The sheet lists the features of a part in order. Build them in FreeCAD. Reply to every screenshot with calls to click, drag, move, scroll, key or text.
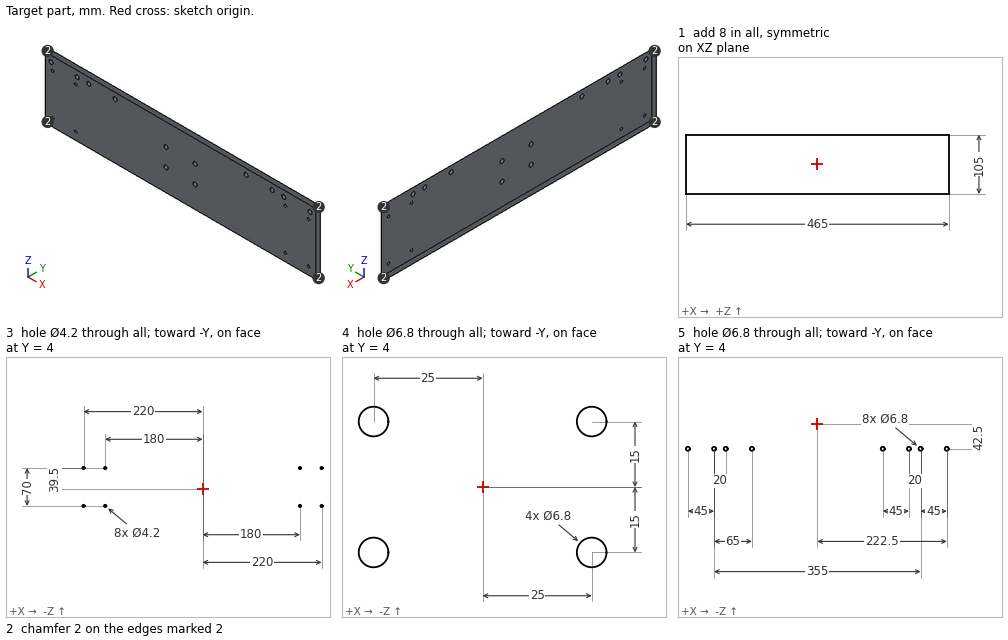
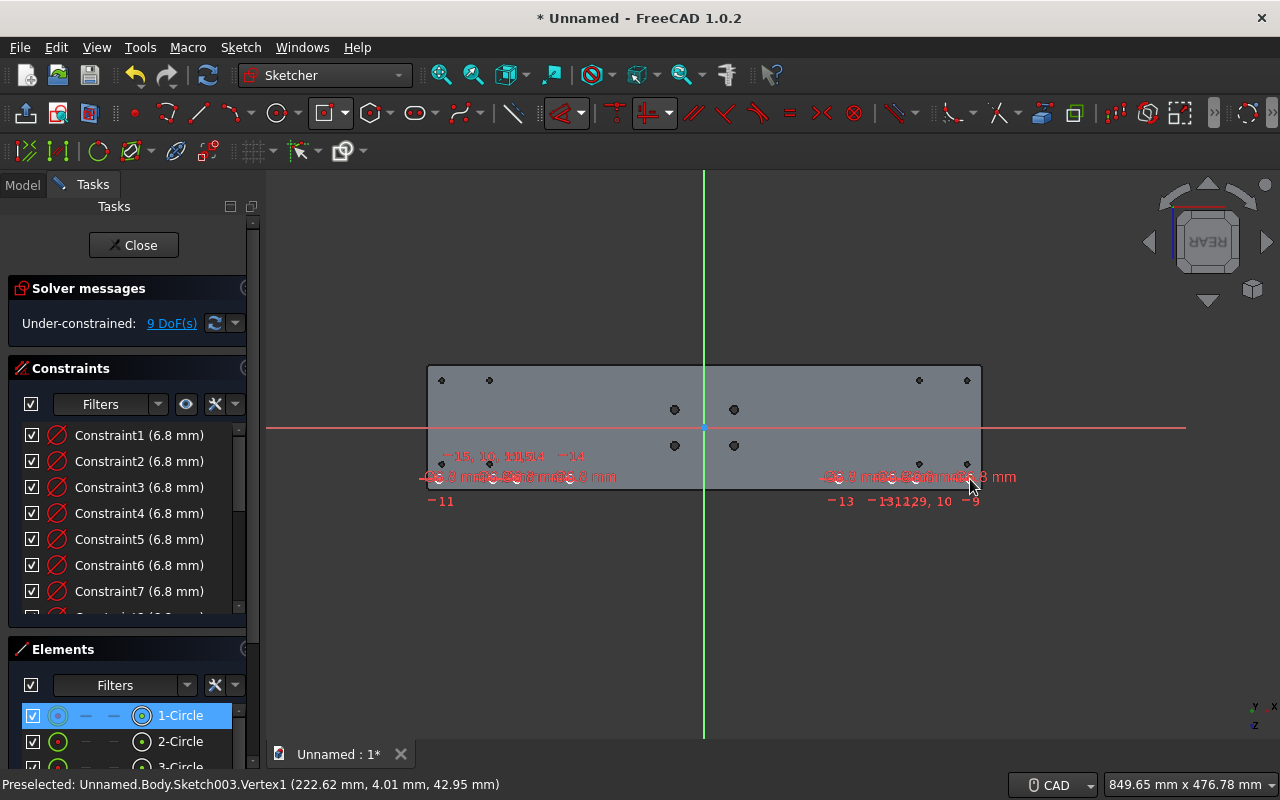
click(916, 479)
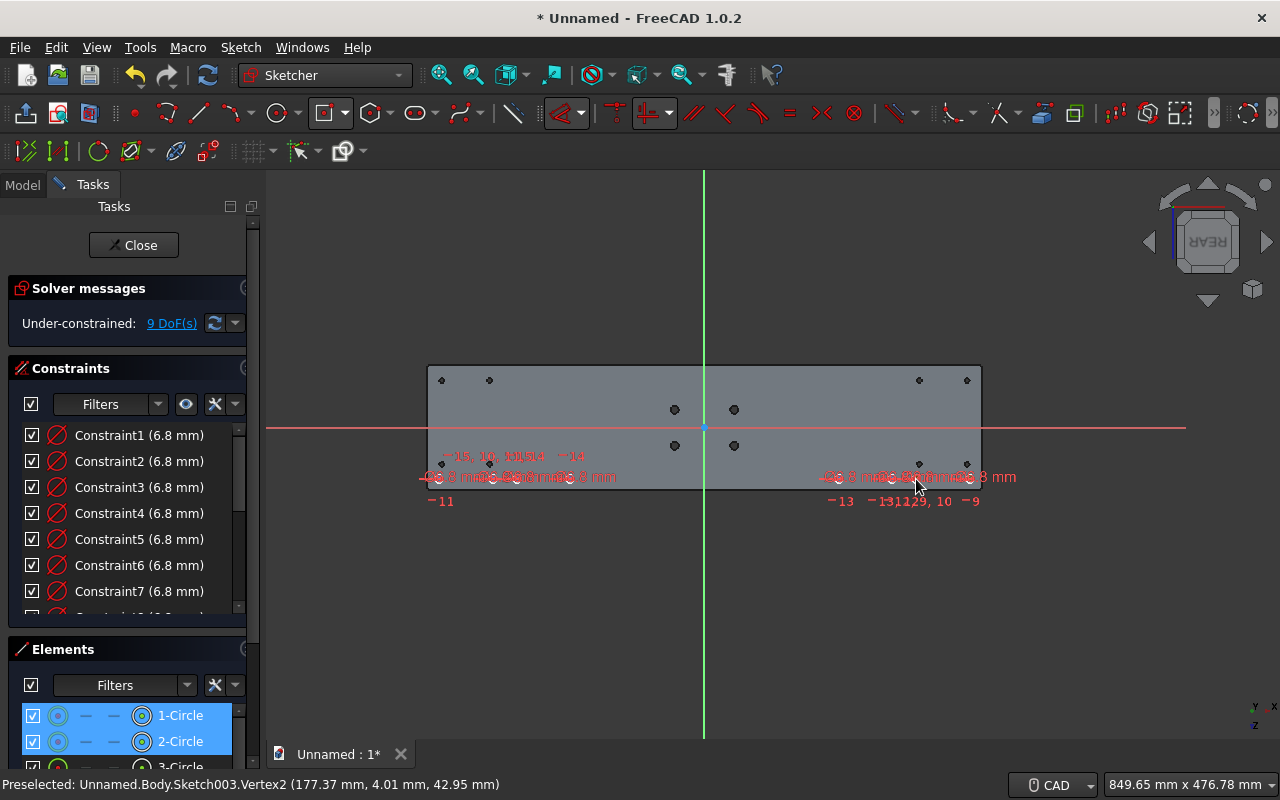
key(l)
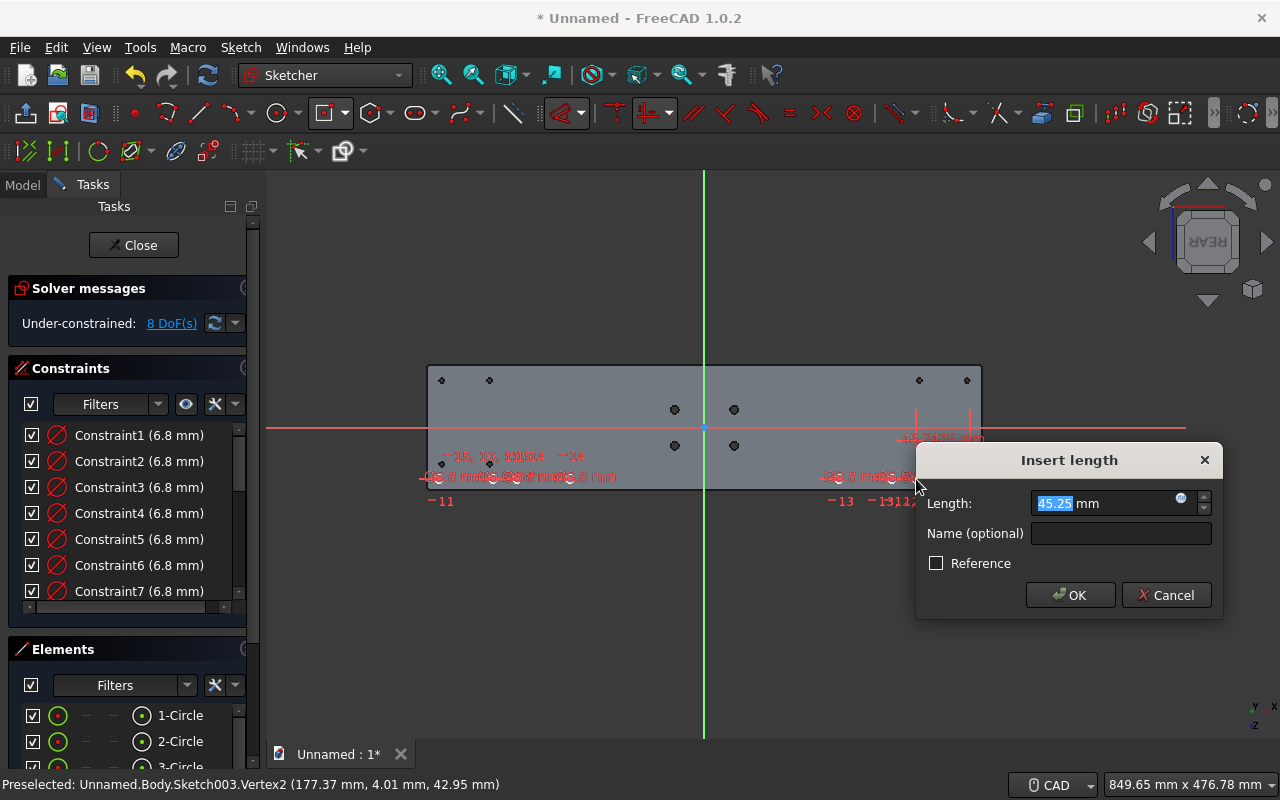
text(45)
key(Return)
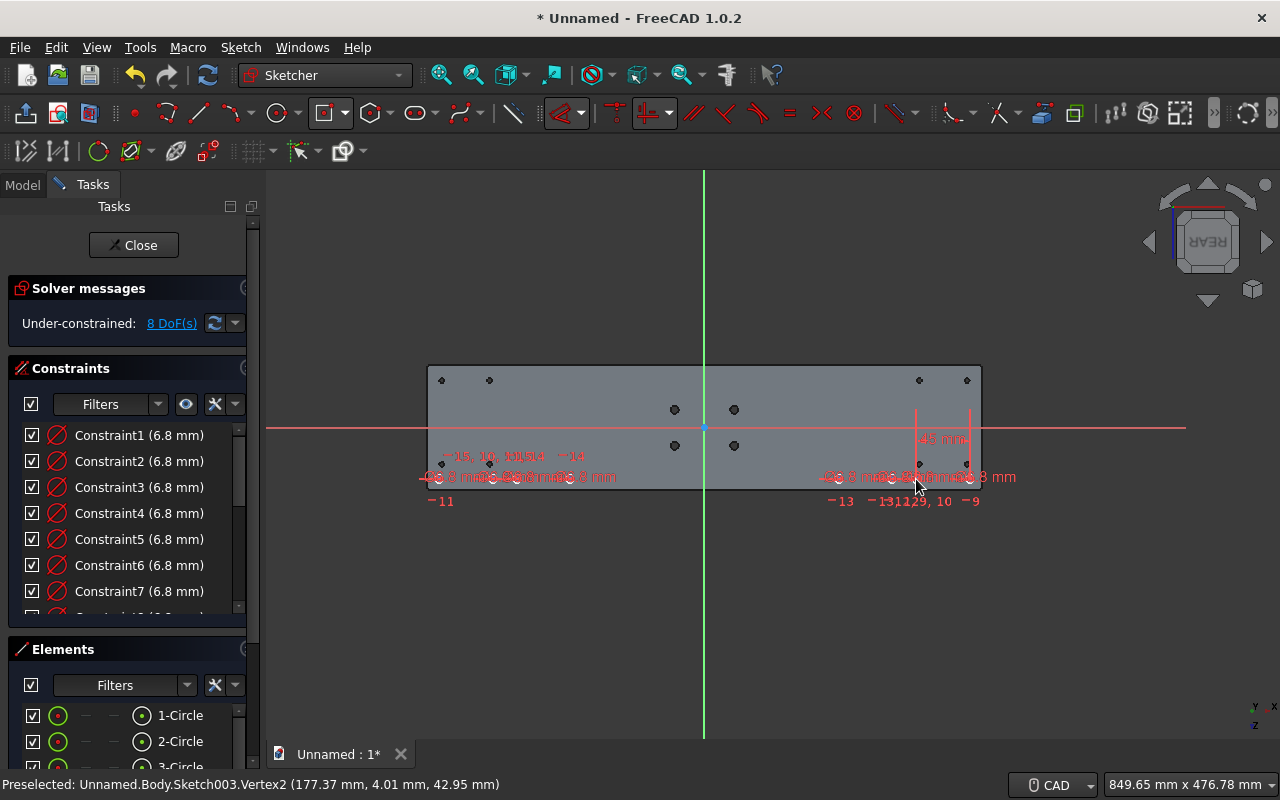
click(493, 479)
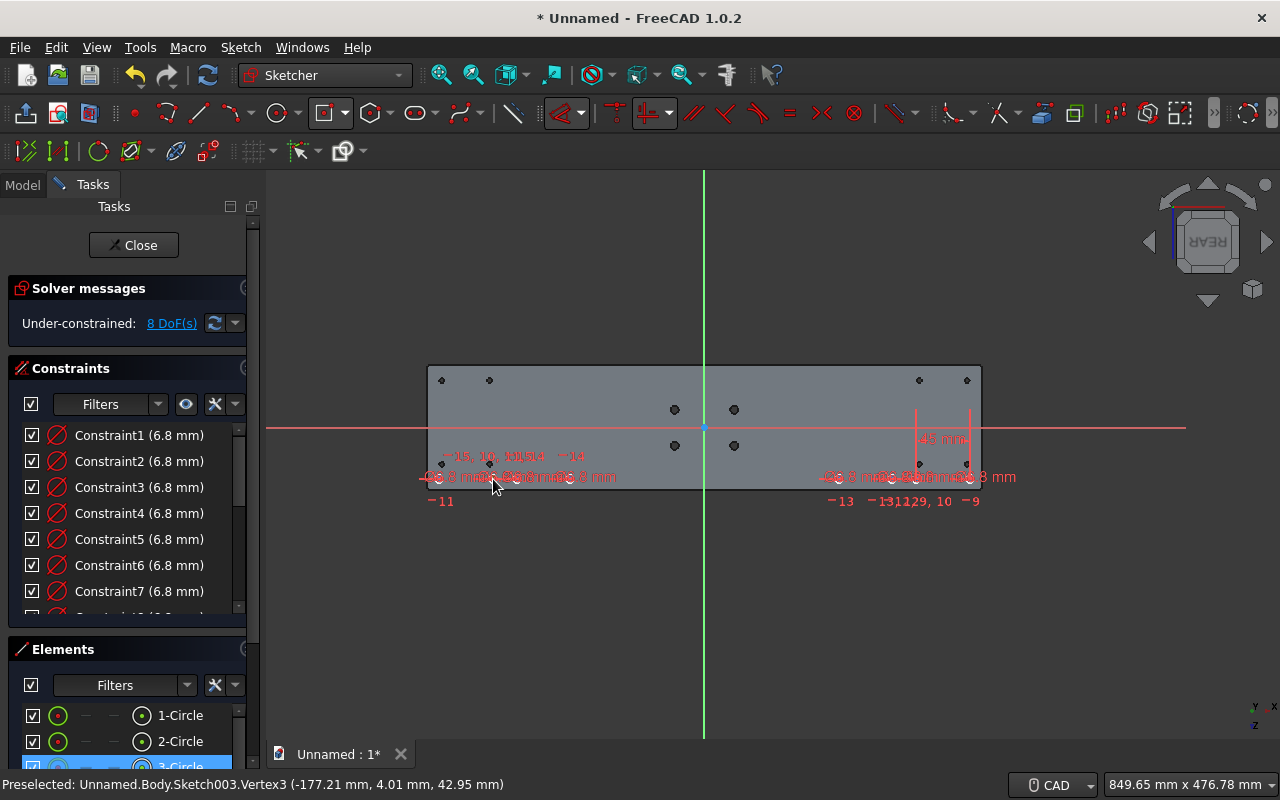
click(439, 479)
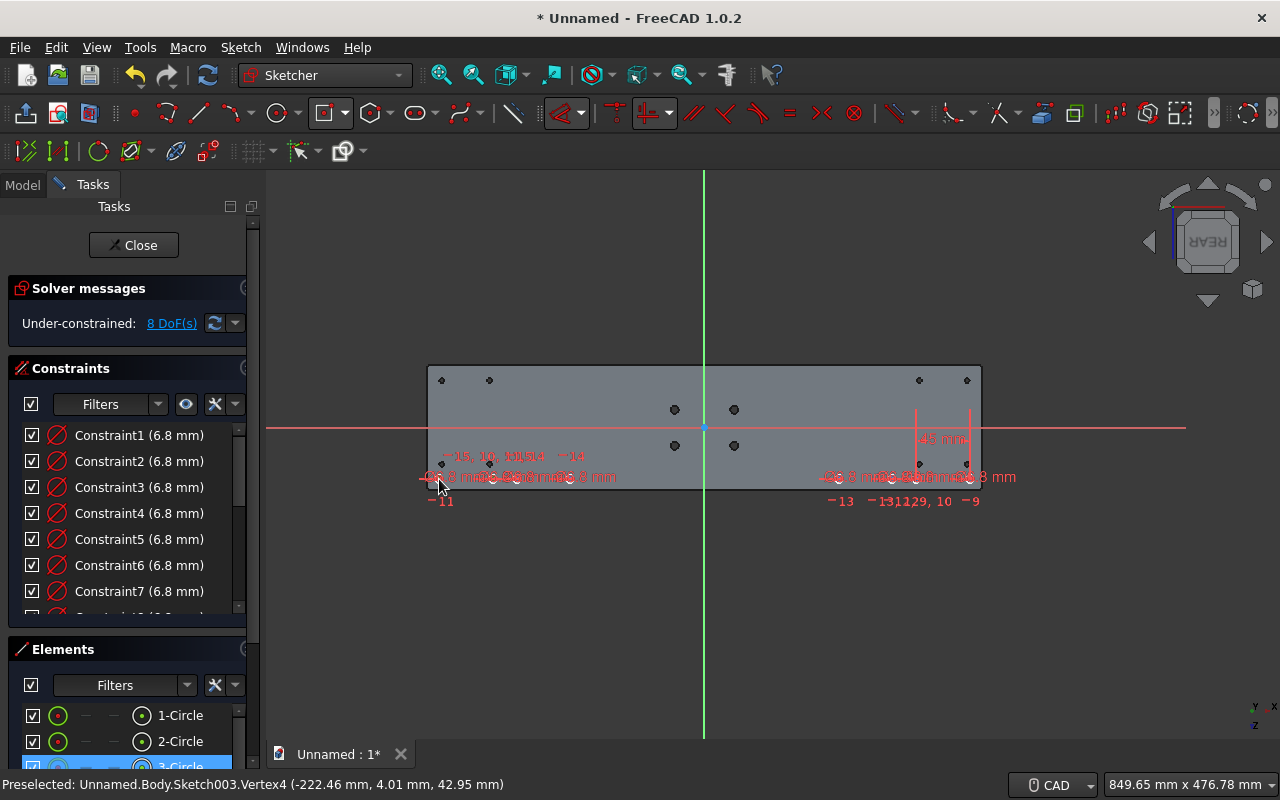
click(584, 114)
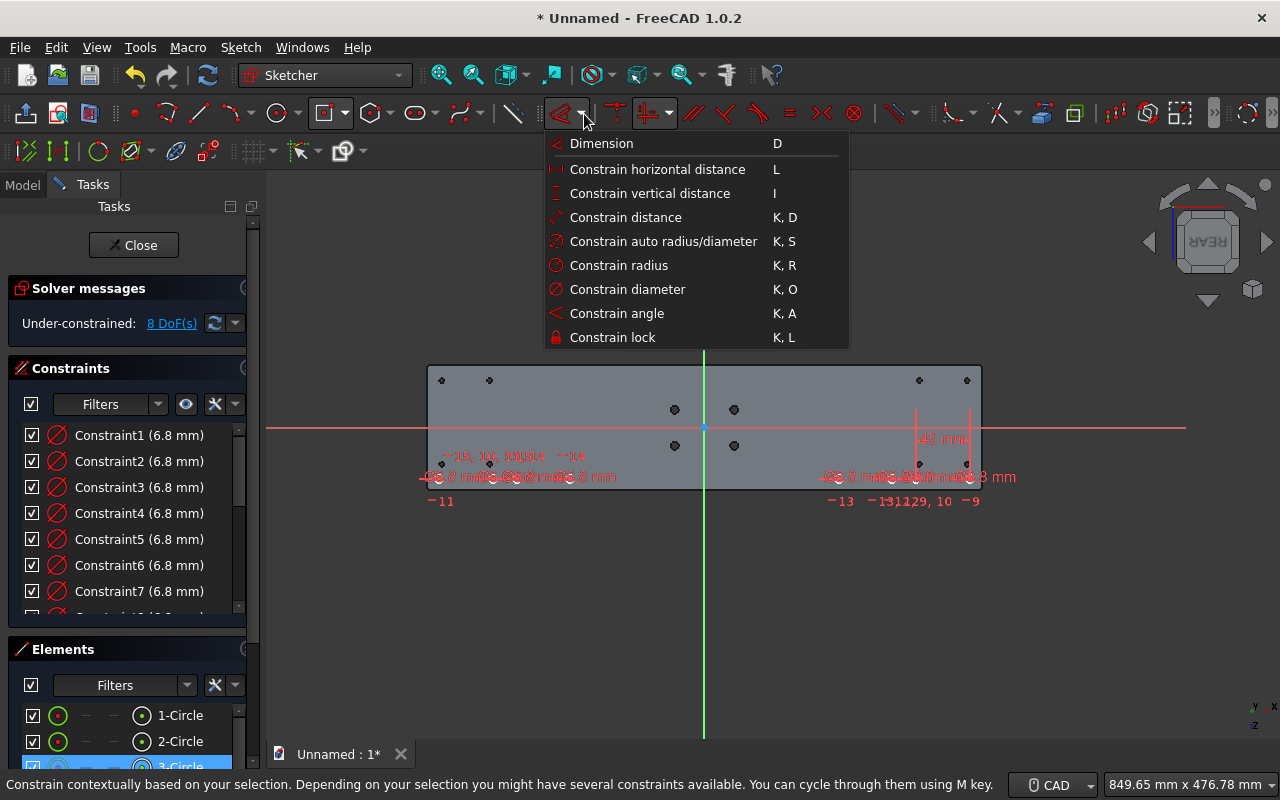
click(697, 169)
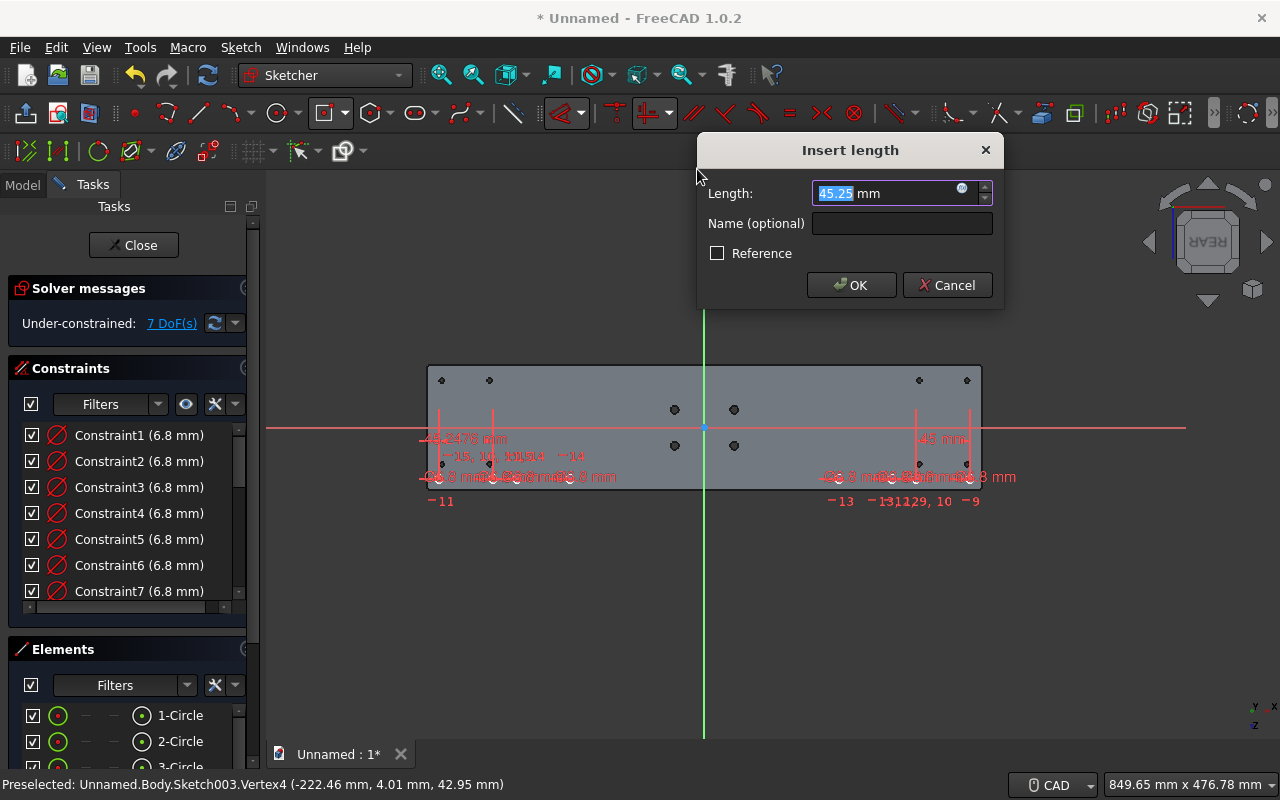
text(45)
key(Return)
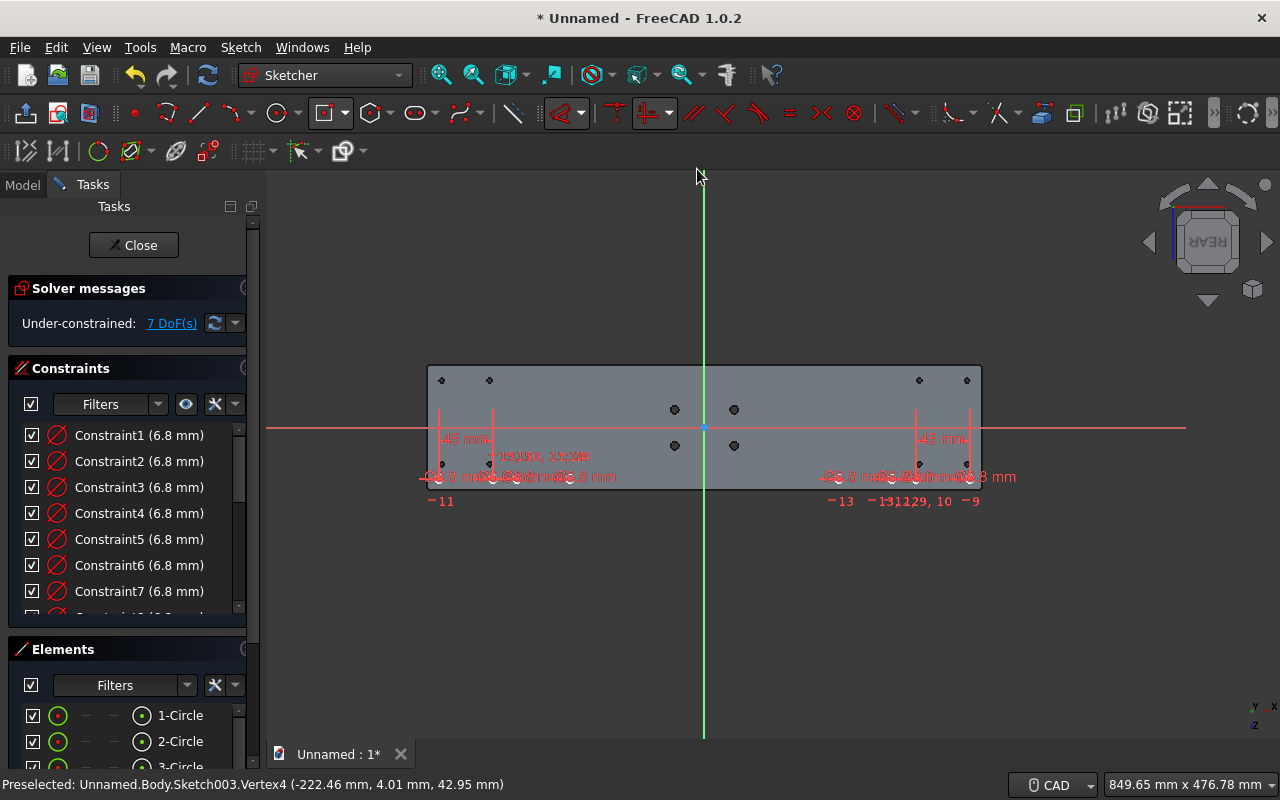
scroll(916, 479, up, 3)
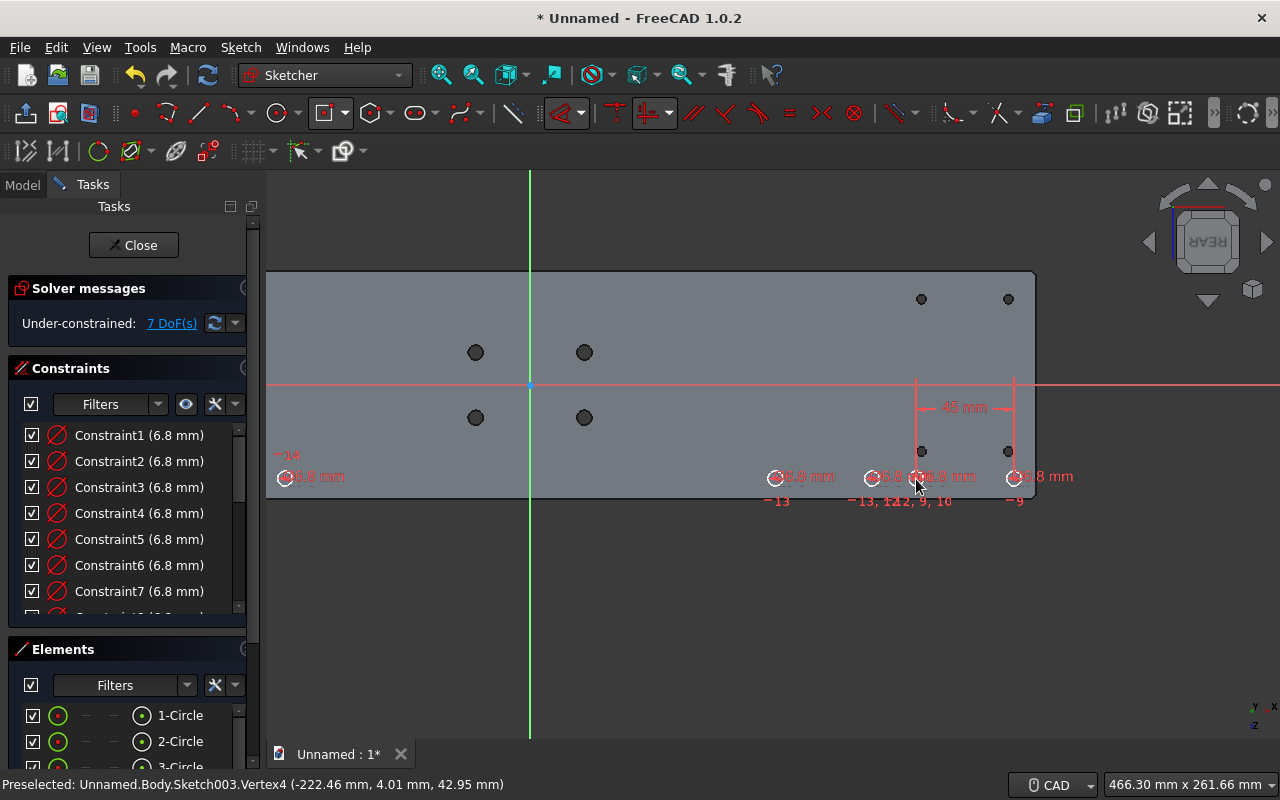
click(916, 479)